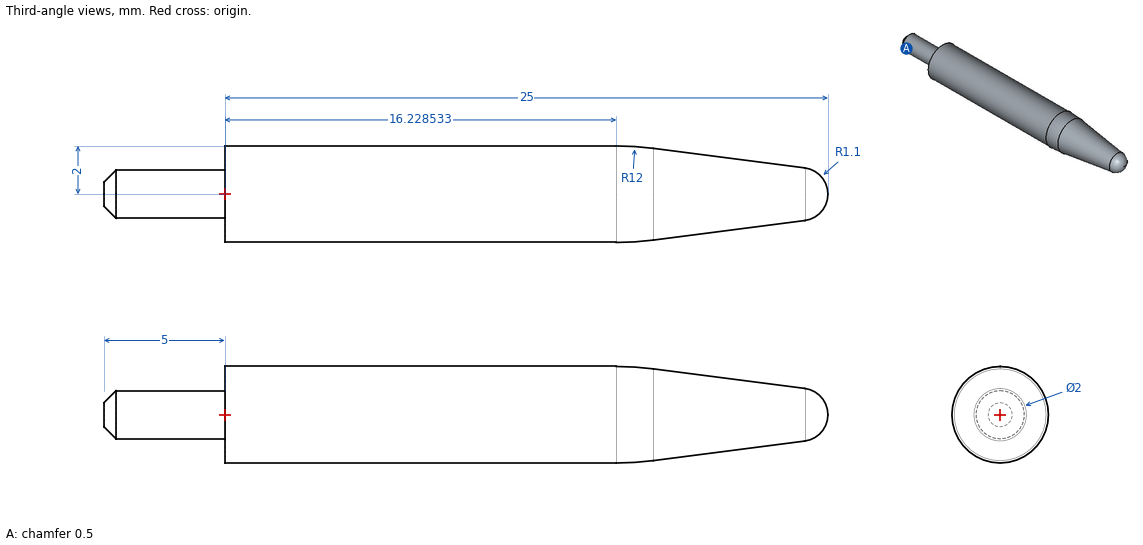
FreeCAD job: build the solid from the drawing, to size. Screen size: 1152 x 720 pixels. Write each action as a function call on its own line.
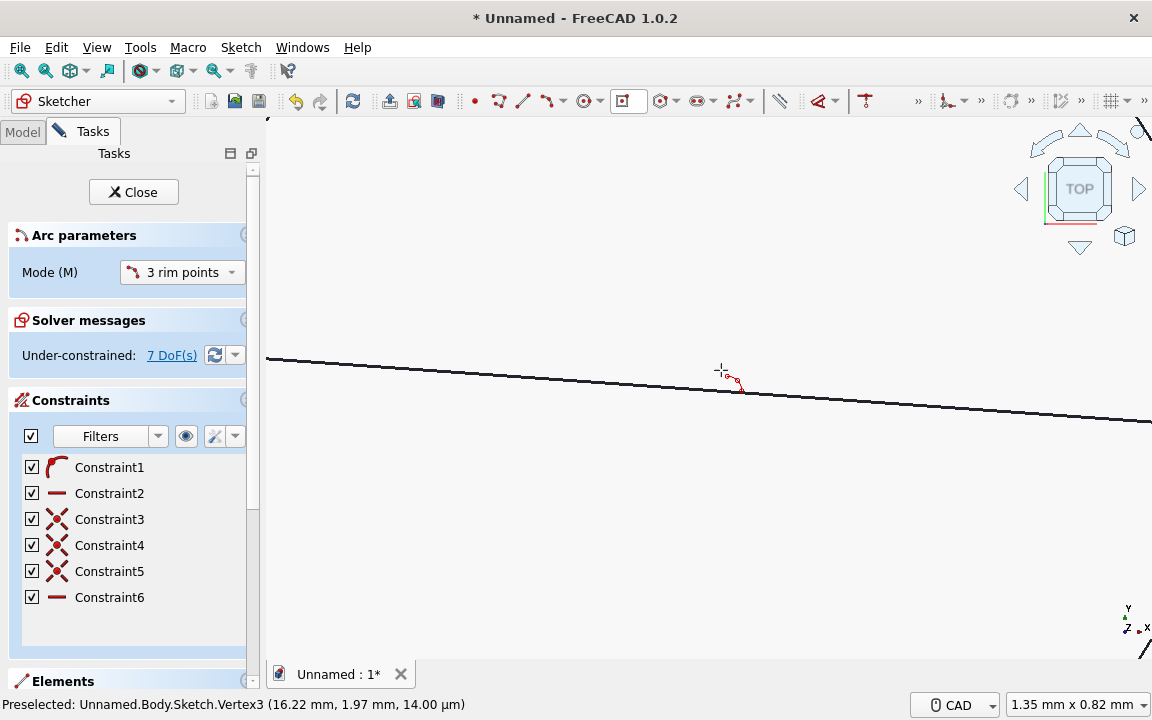
click(705, 349)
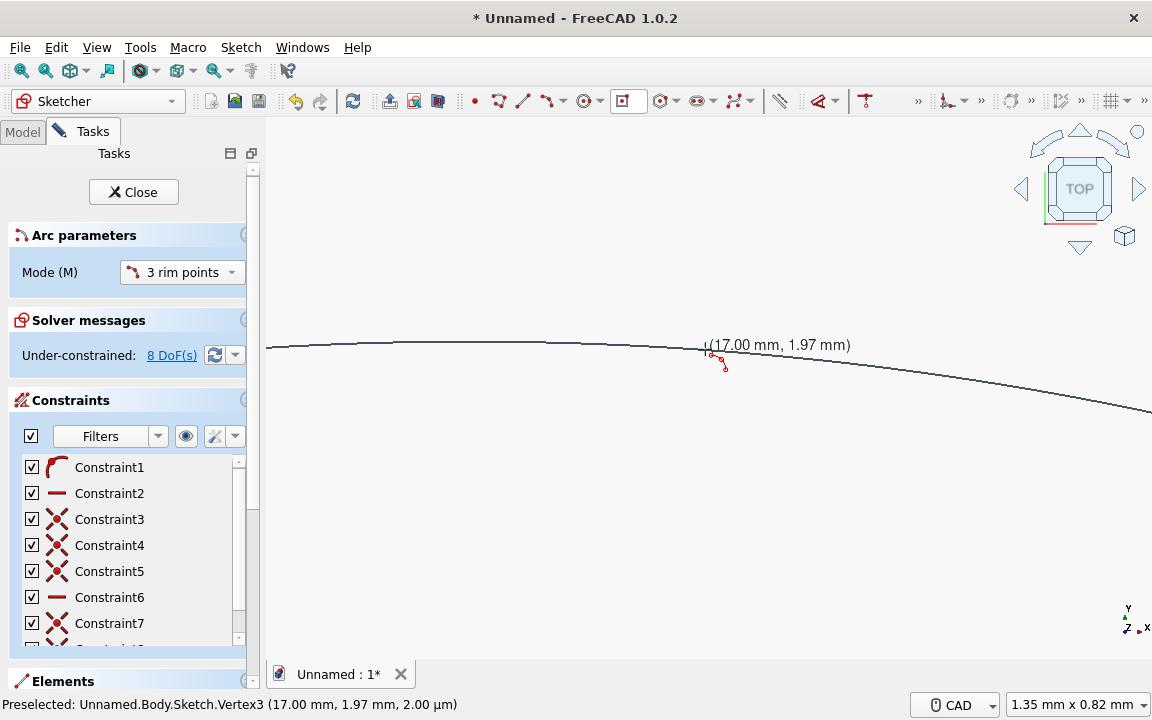
scroll(741, 367, down, 17)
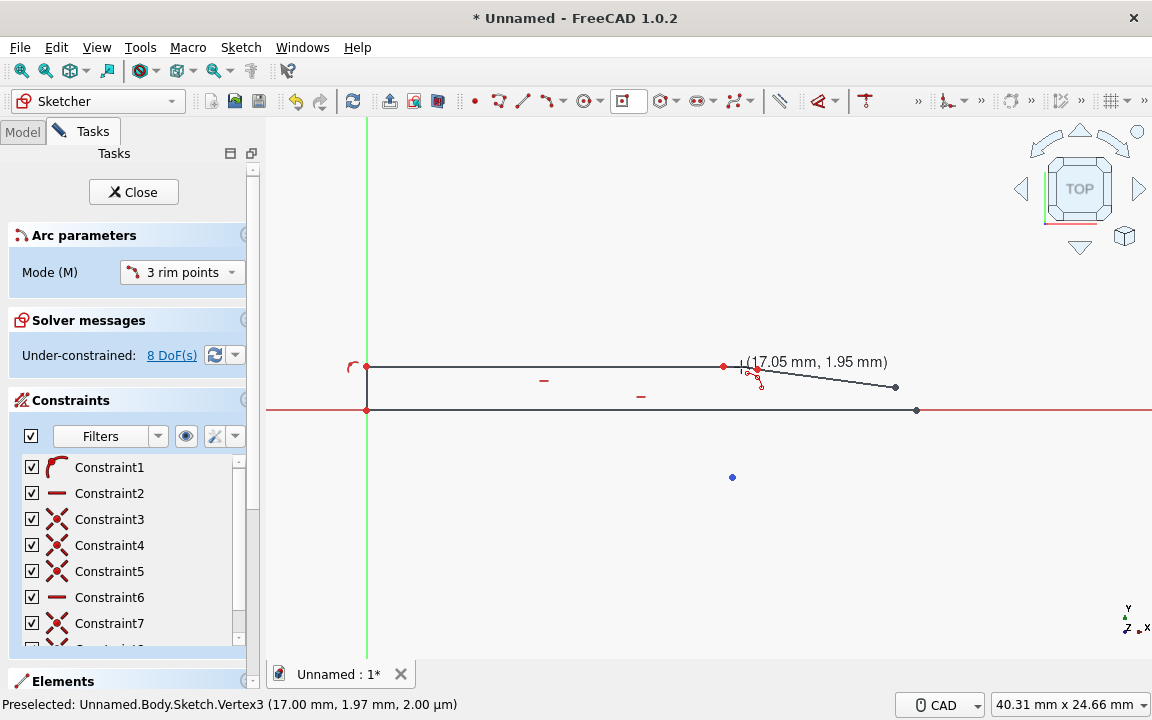
click(916, 399)
click(895, 388)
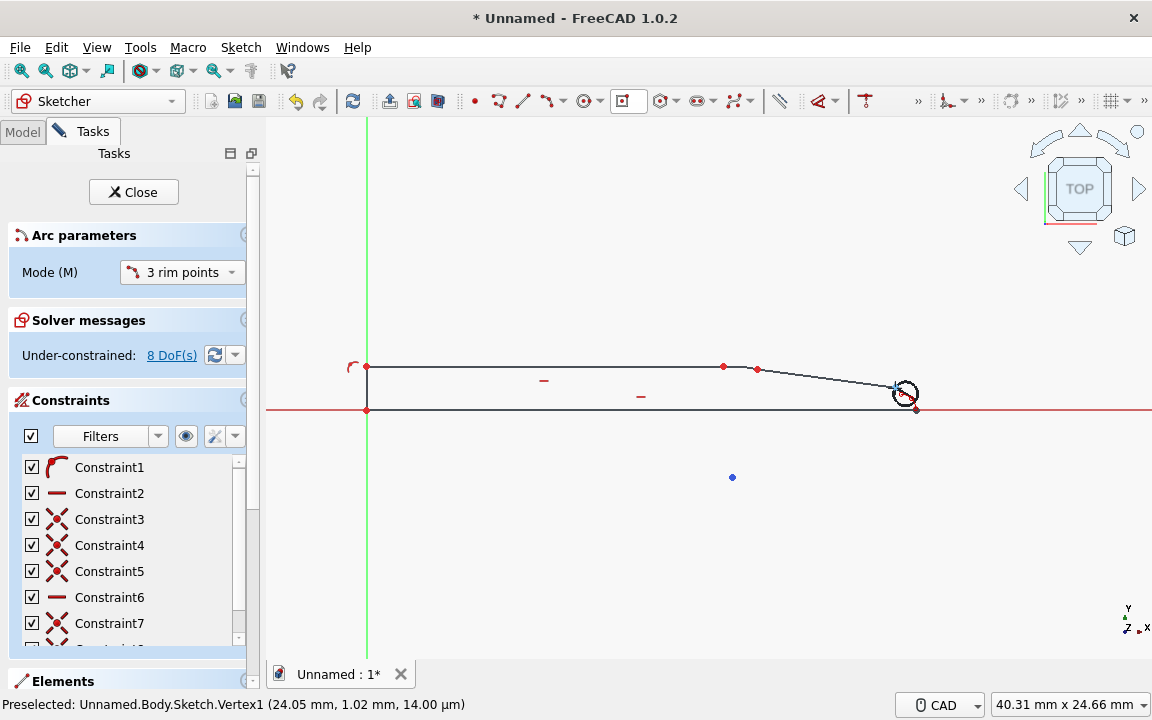
scroll(910, 394, up, 5)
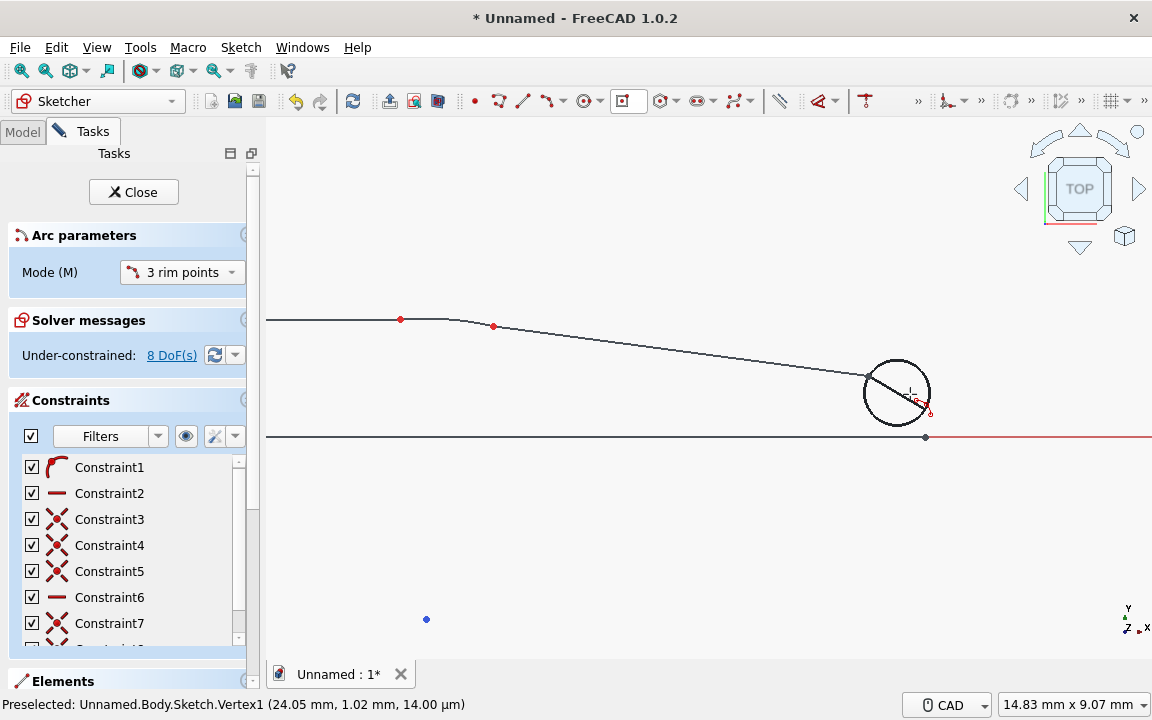
click(909, 394)
key(Escape)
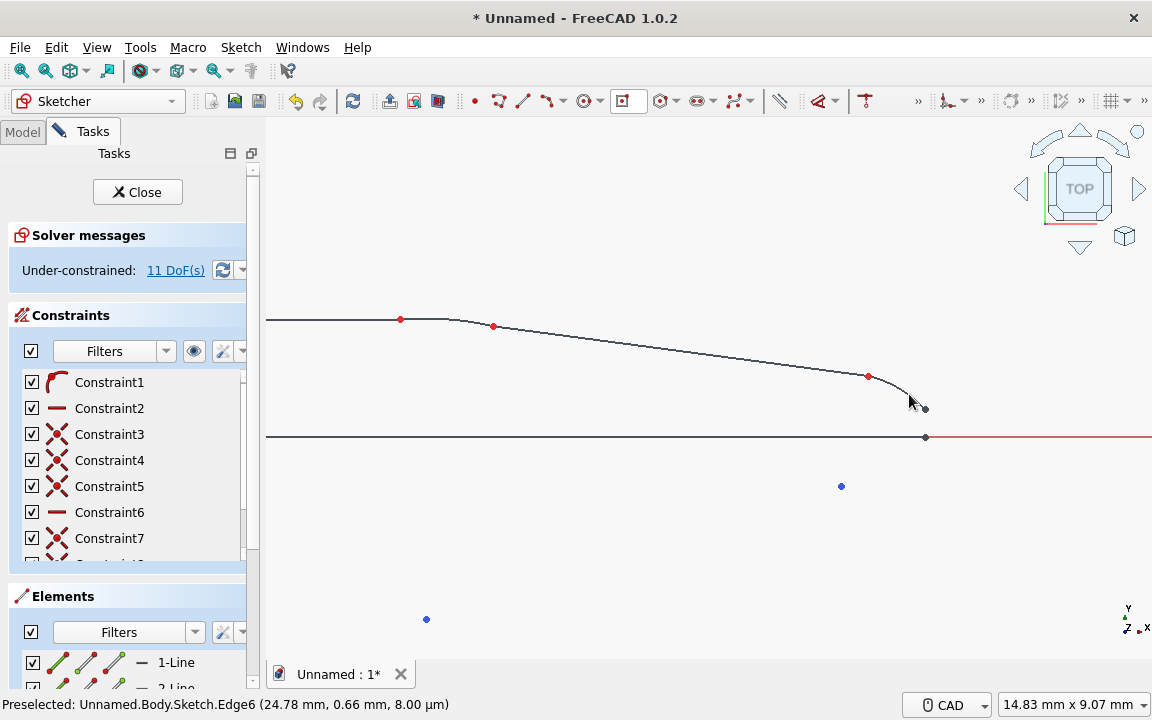
click(756, 361)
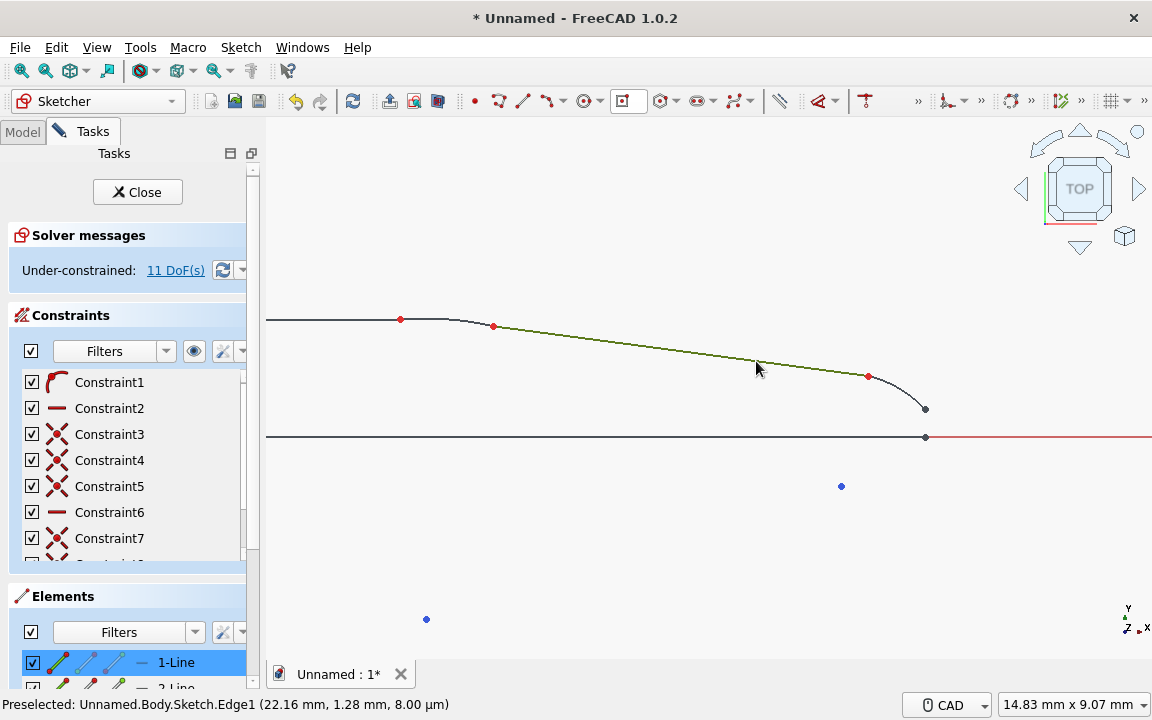
click(466, 321)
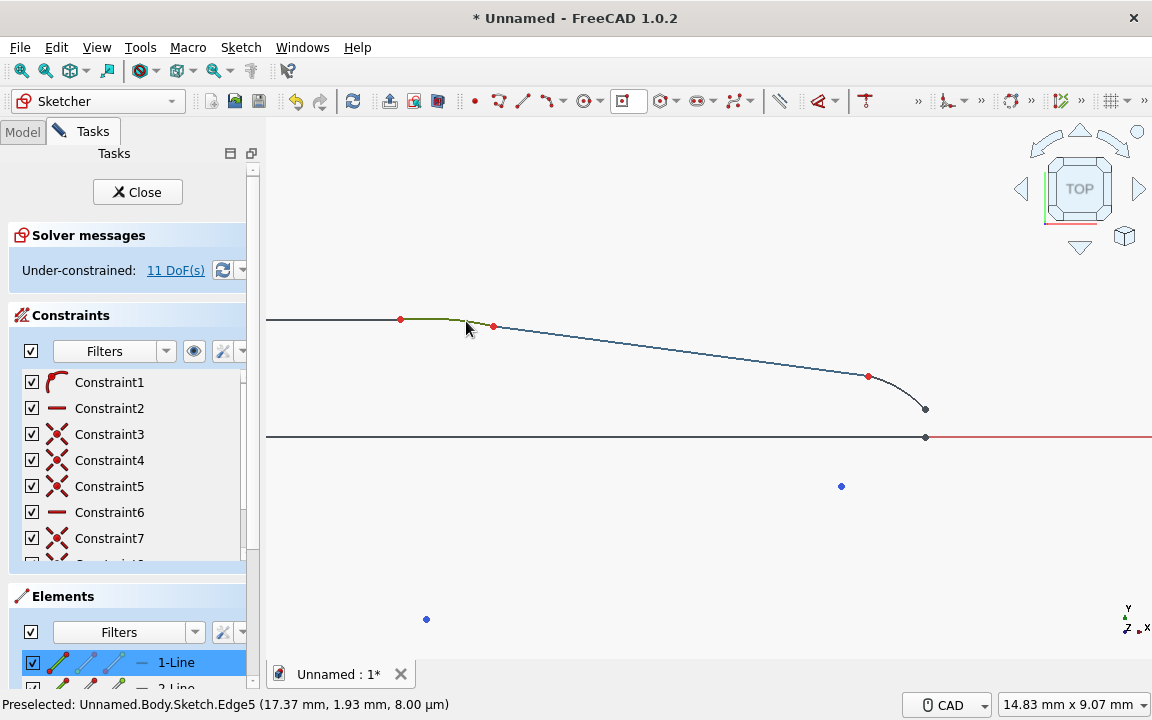
key(t)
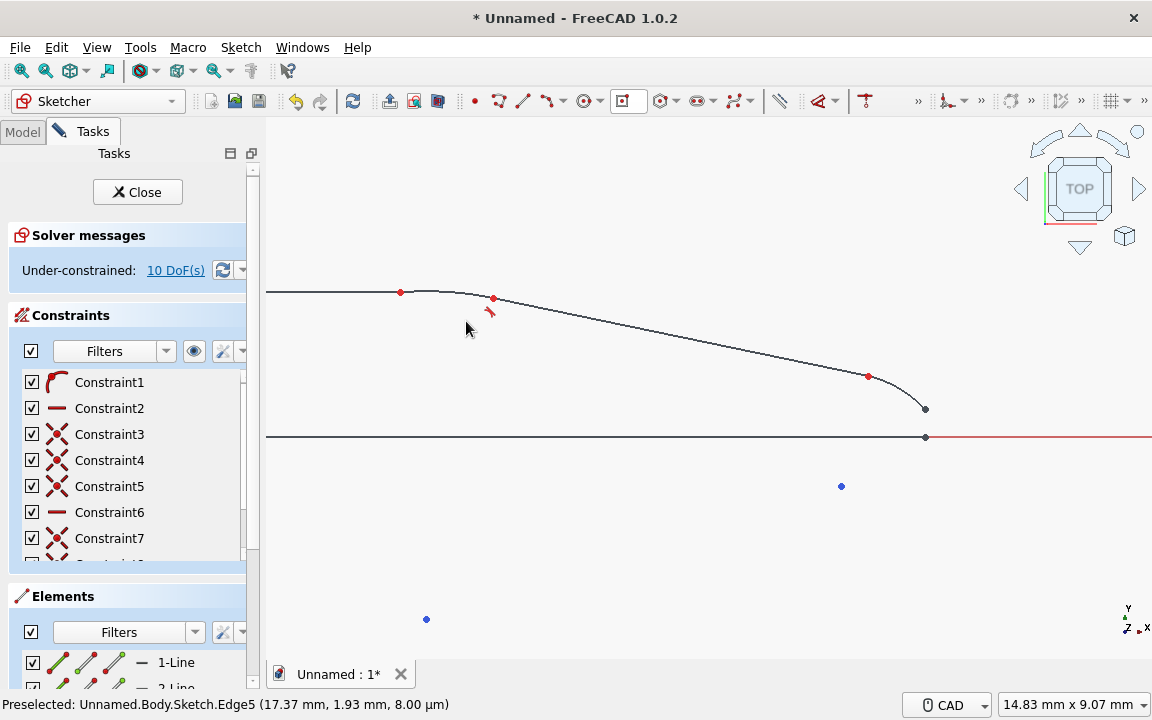
click(756, 353)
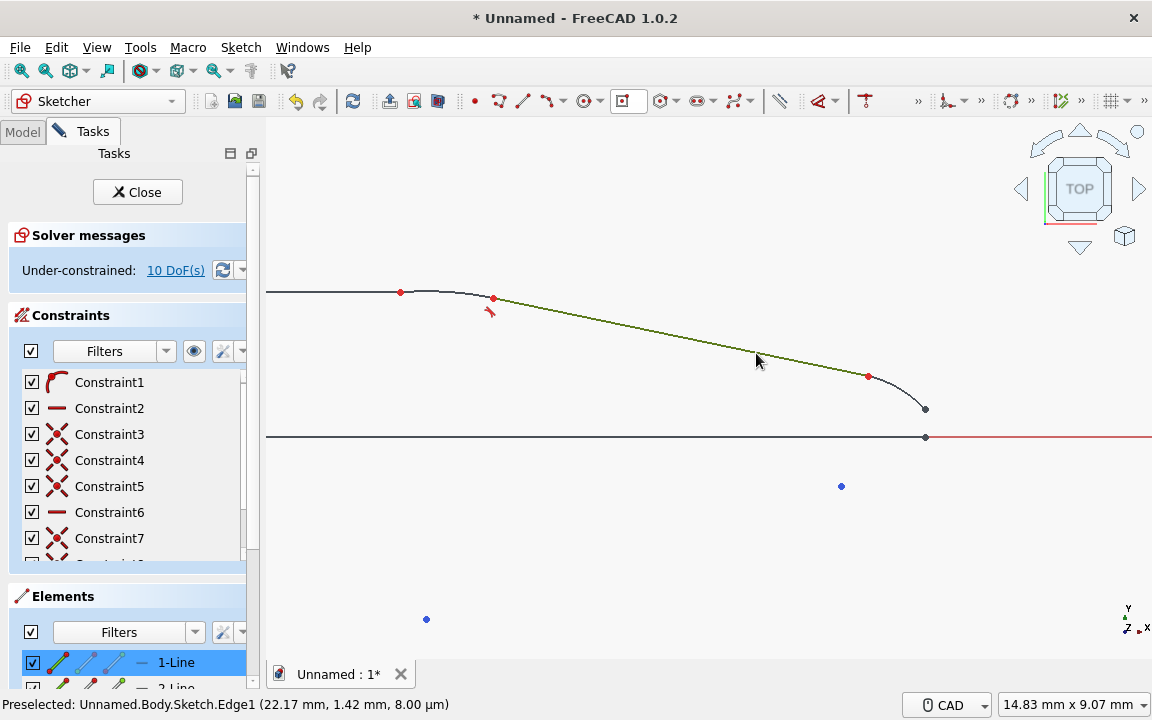
click(910, 396)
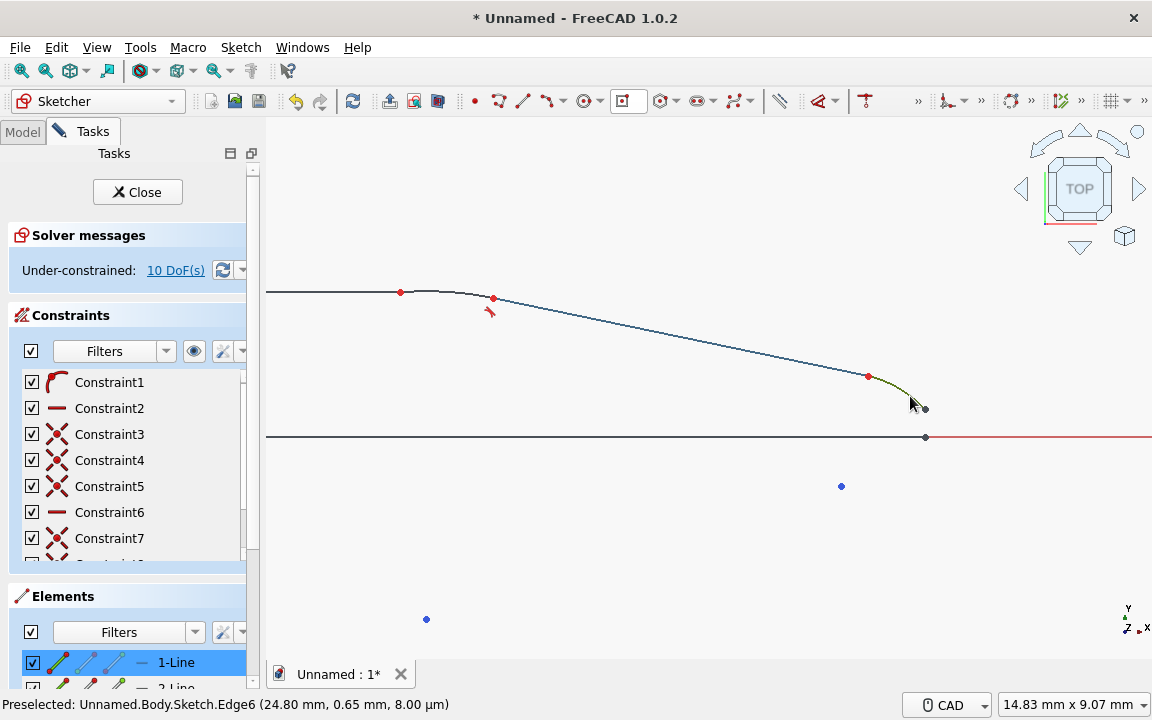
key(t)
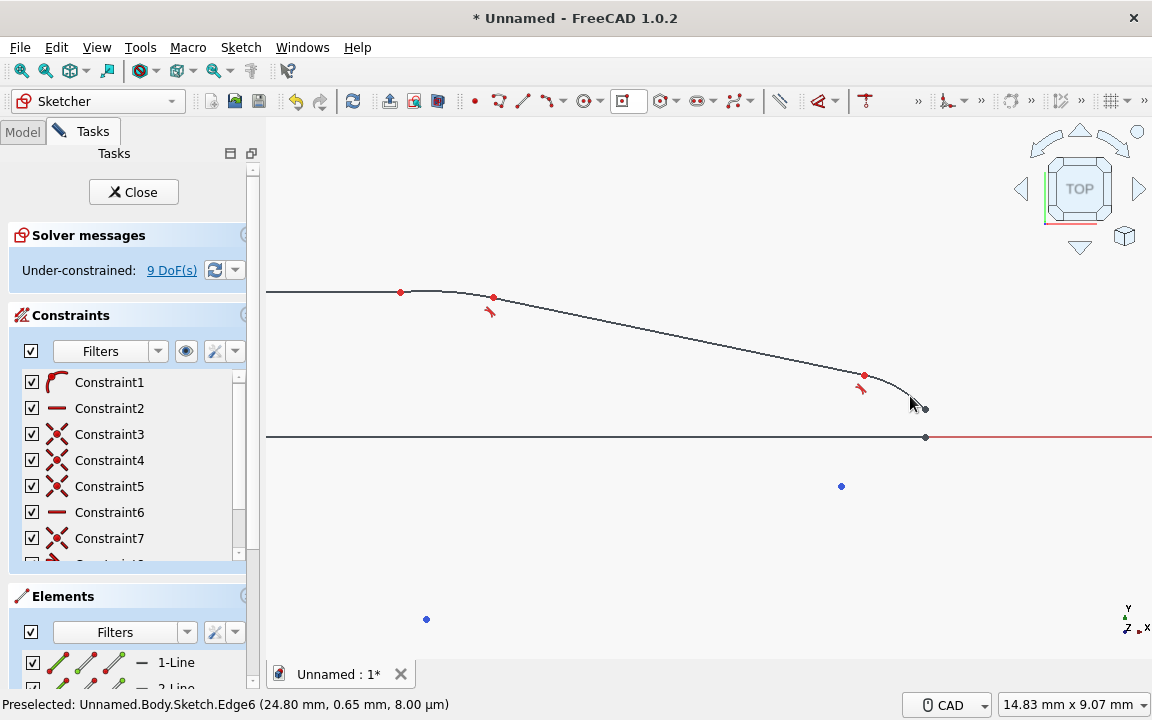
scroll(840, 392, down, 6)